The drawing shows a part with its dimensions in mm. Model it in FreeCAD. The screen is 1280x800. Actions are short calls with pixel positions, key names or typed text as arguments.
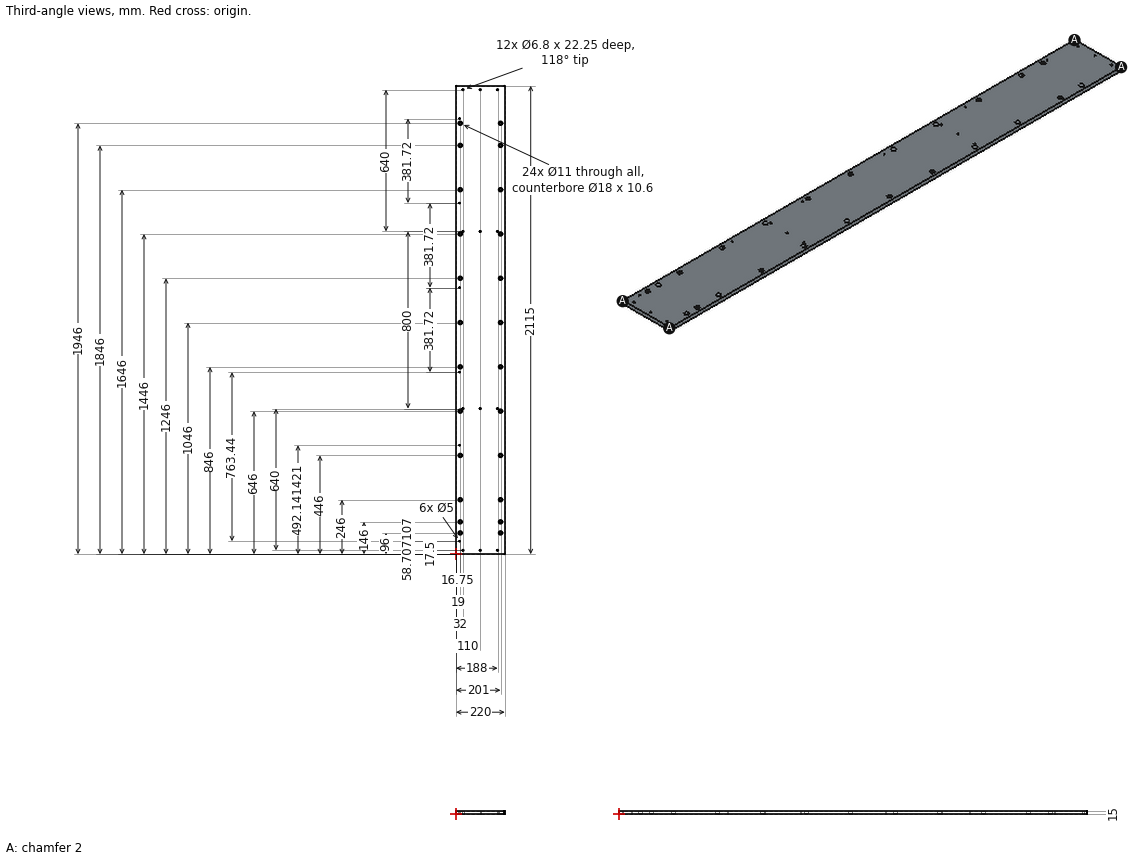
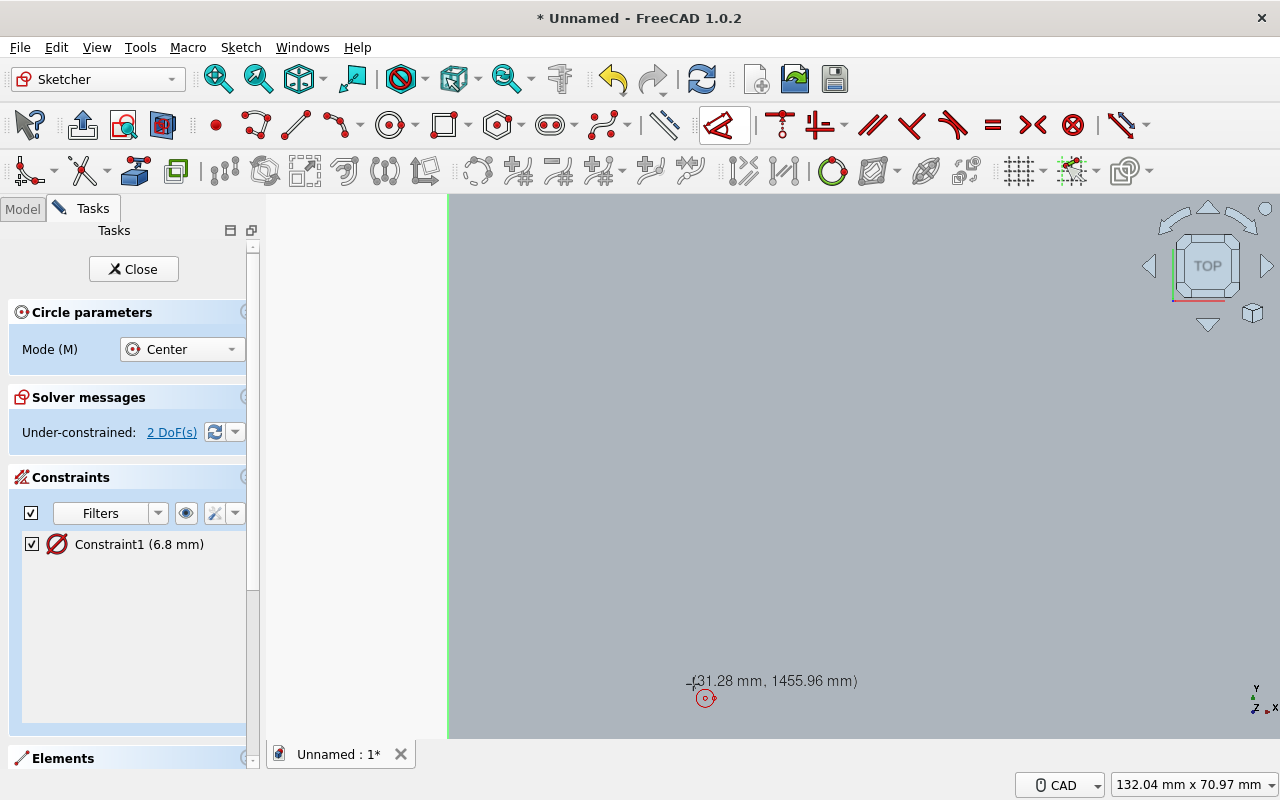
scroll(704, 466, down, 15)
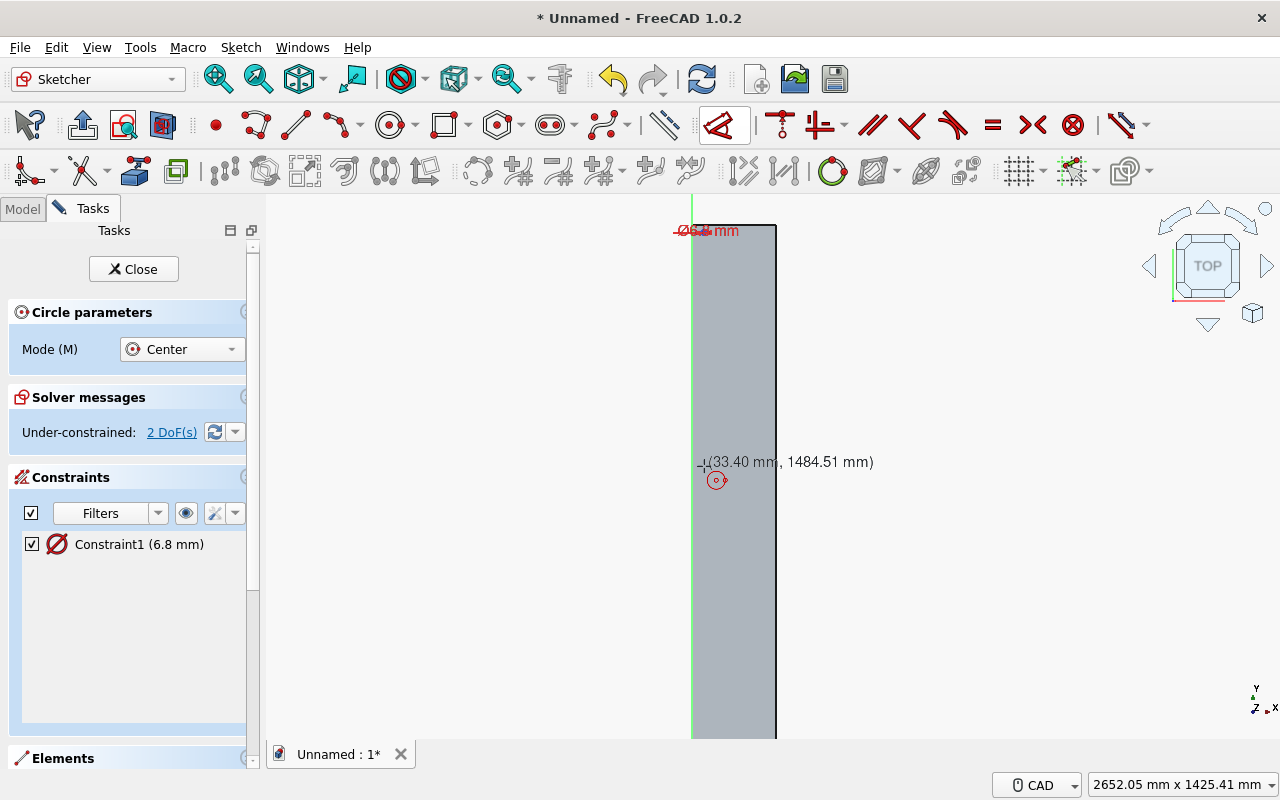
scroll(685, 331, down, 4)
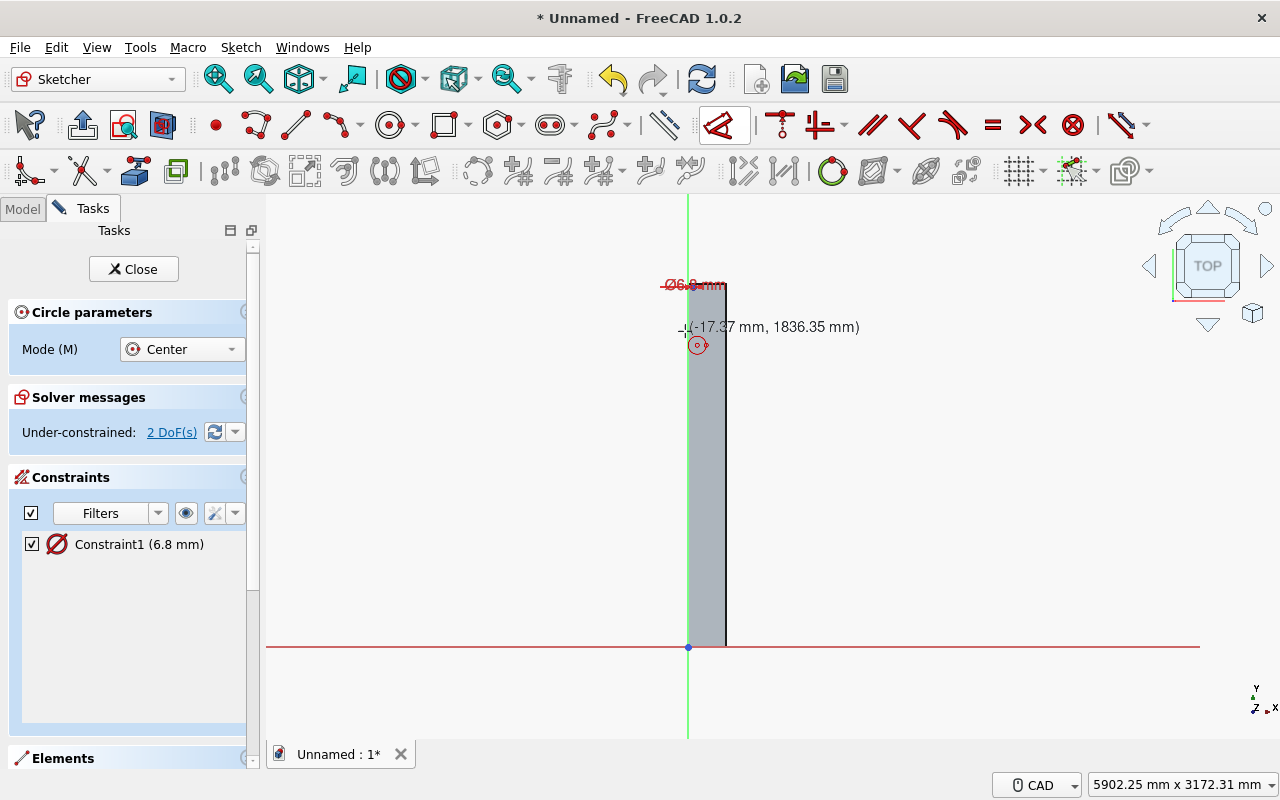
scroll(694, 397, up, 6)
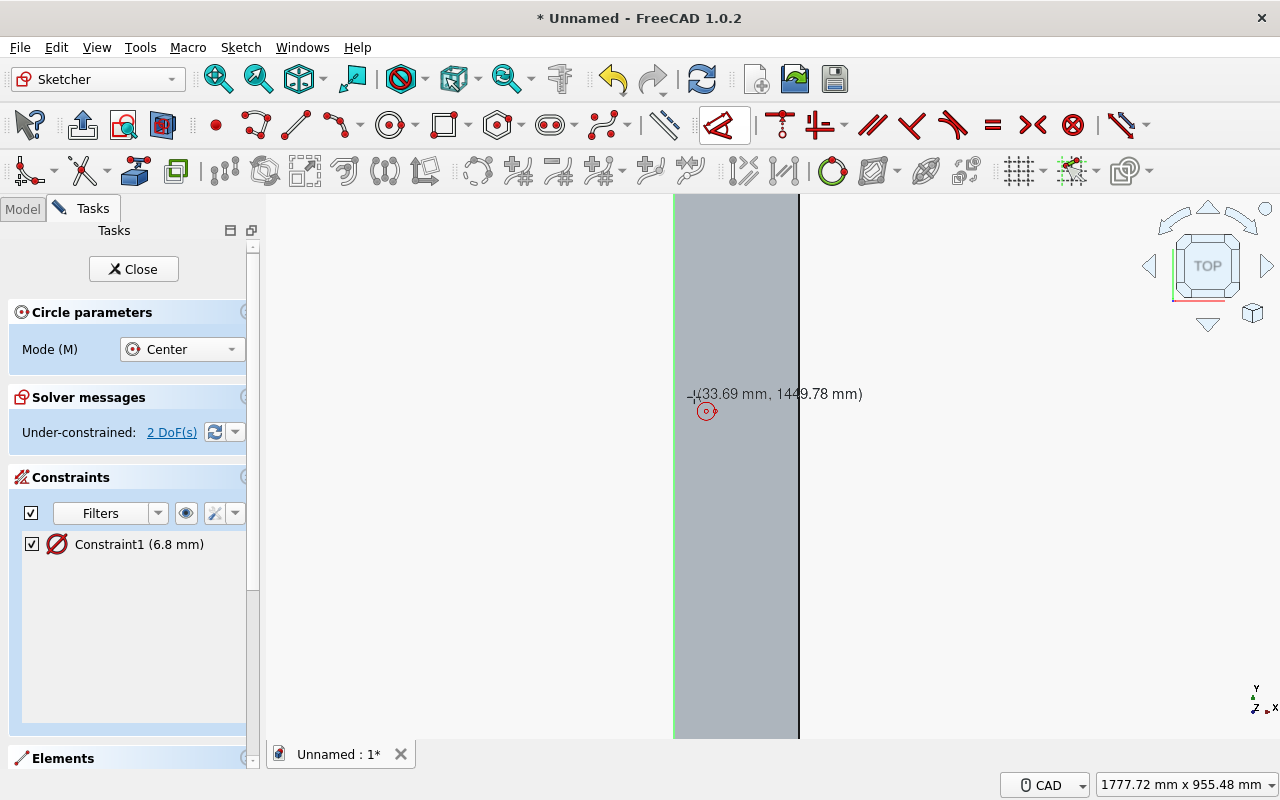
click(692, 395)
move(693, 394)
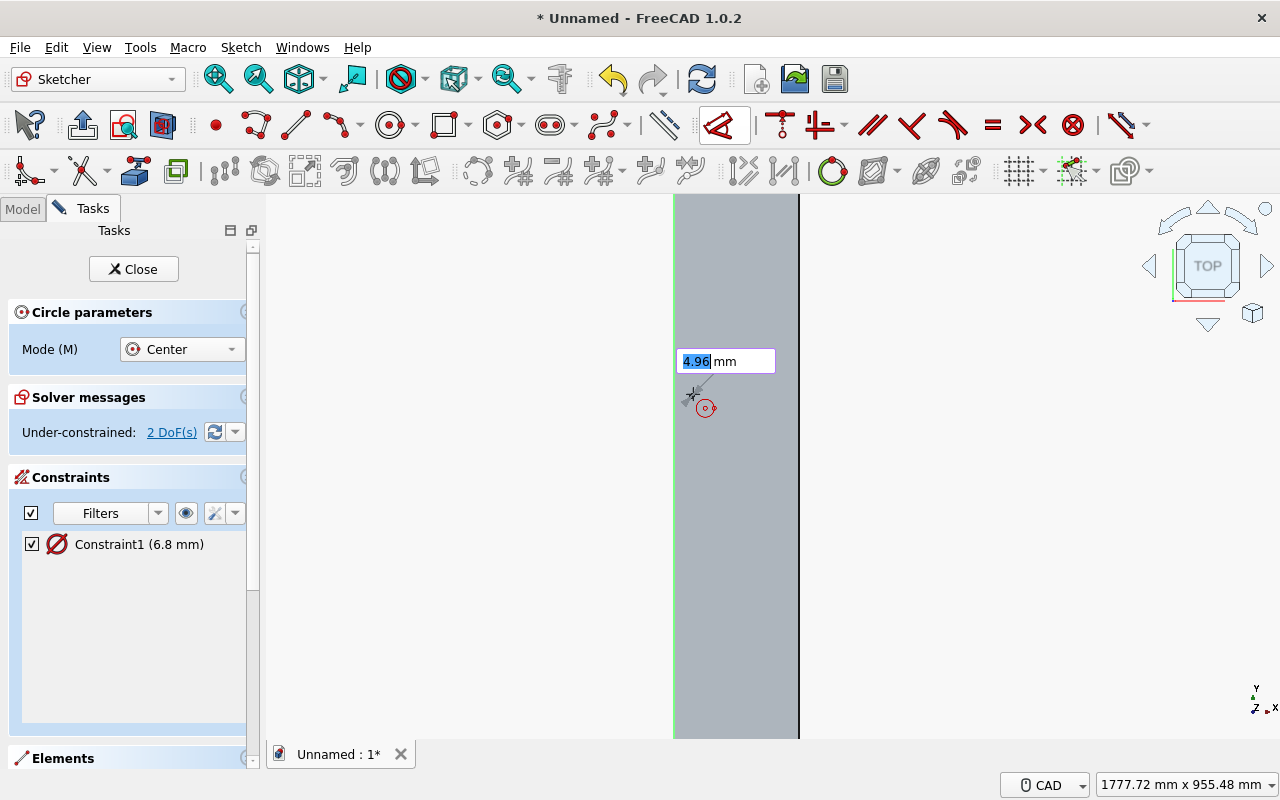
text(6.8)
key(Return)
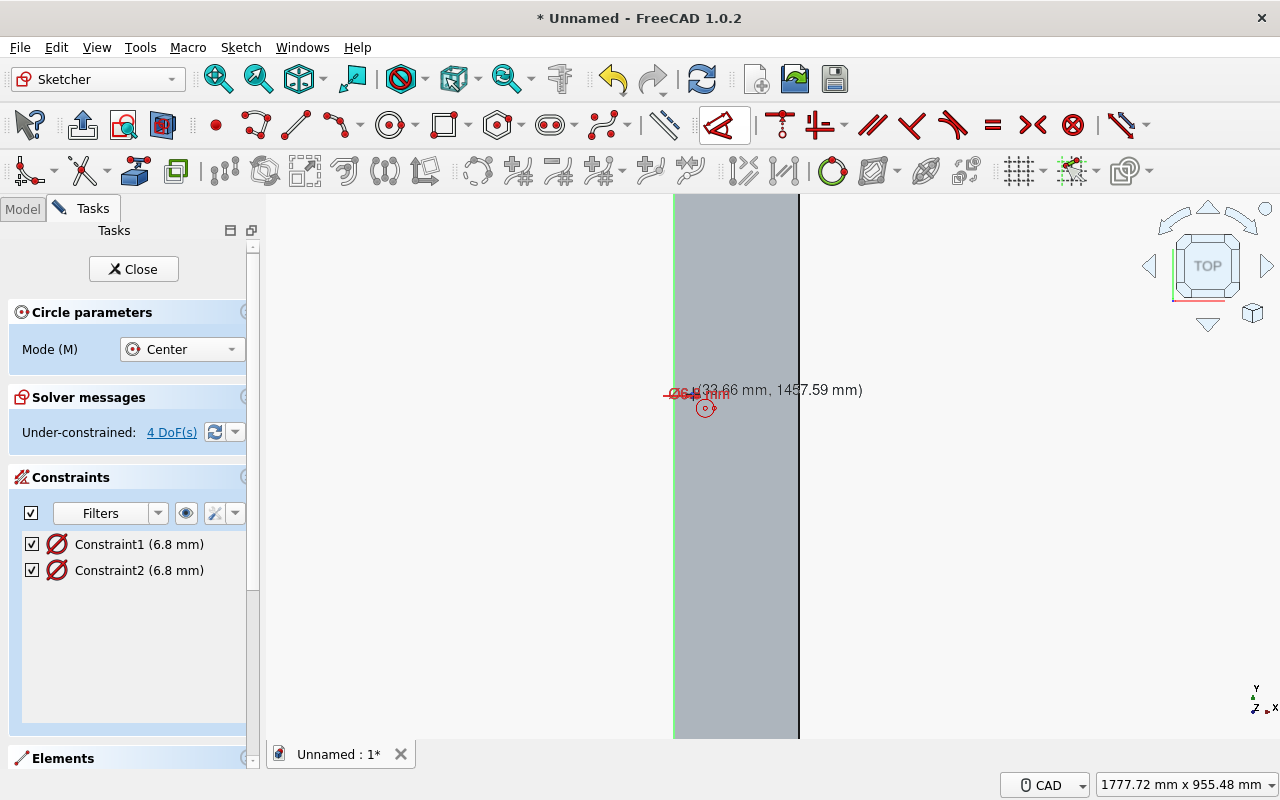
scroll(694, 397, down, 6)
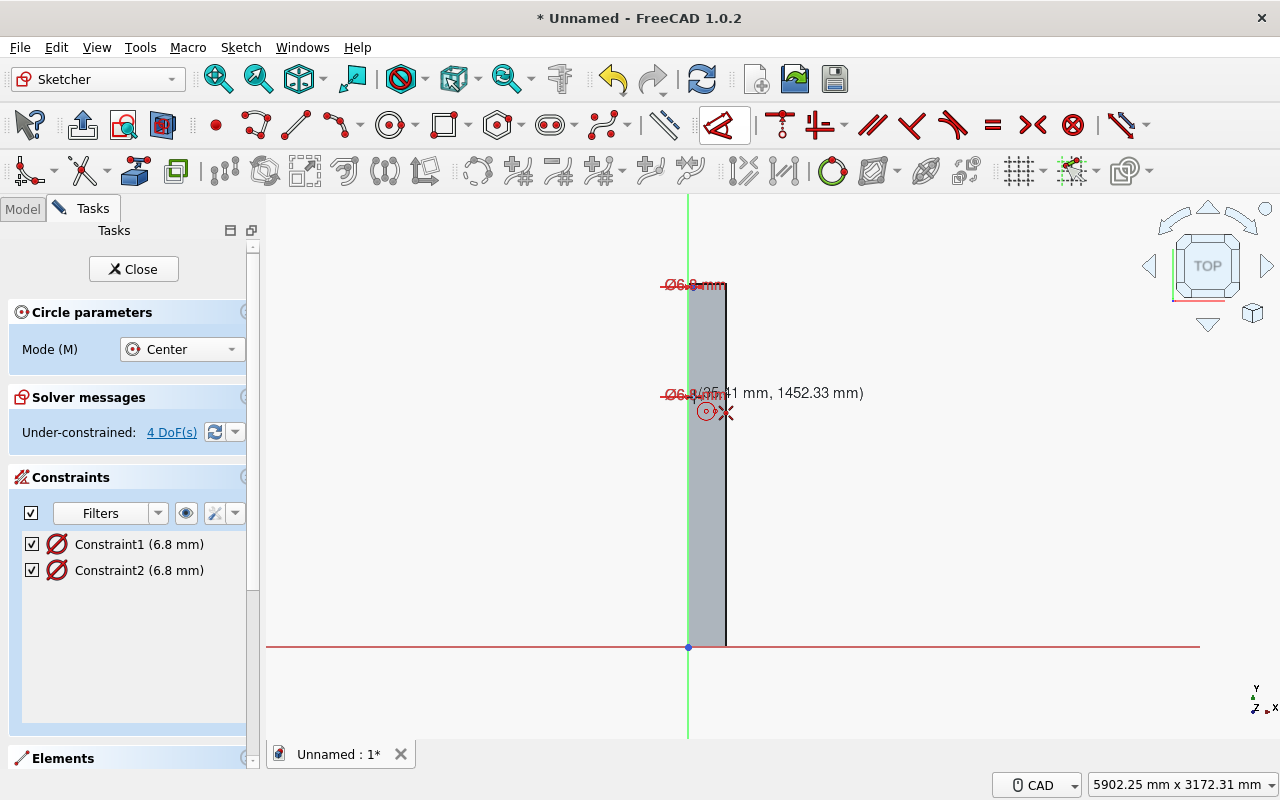
scroll(694, 534, up, 19)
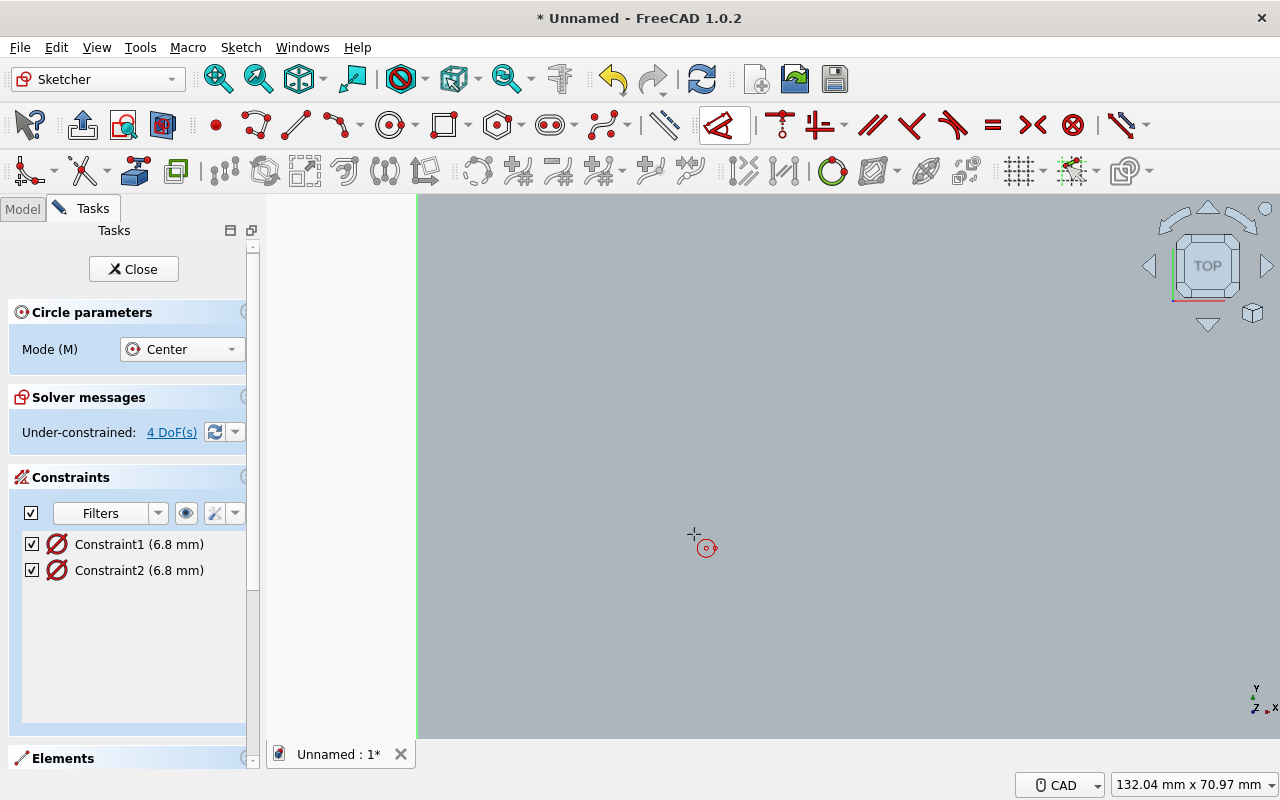
scroll(704, 466, down, 15)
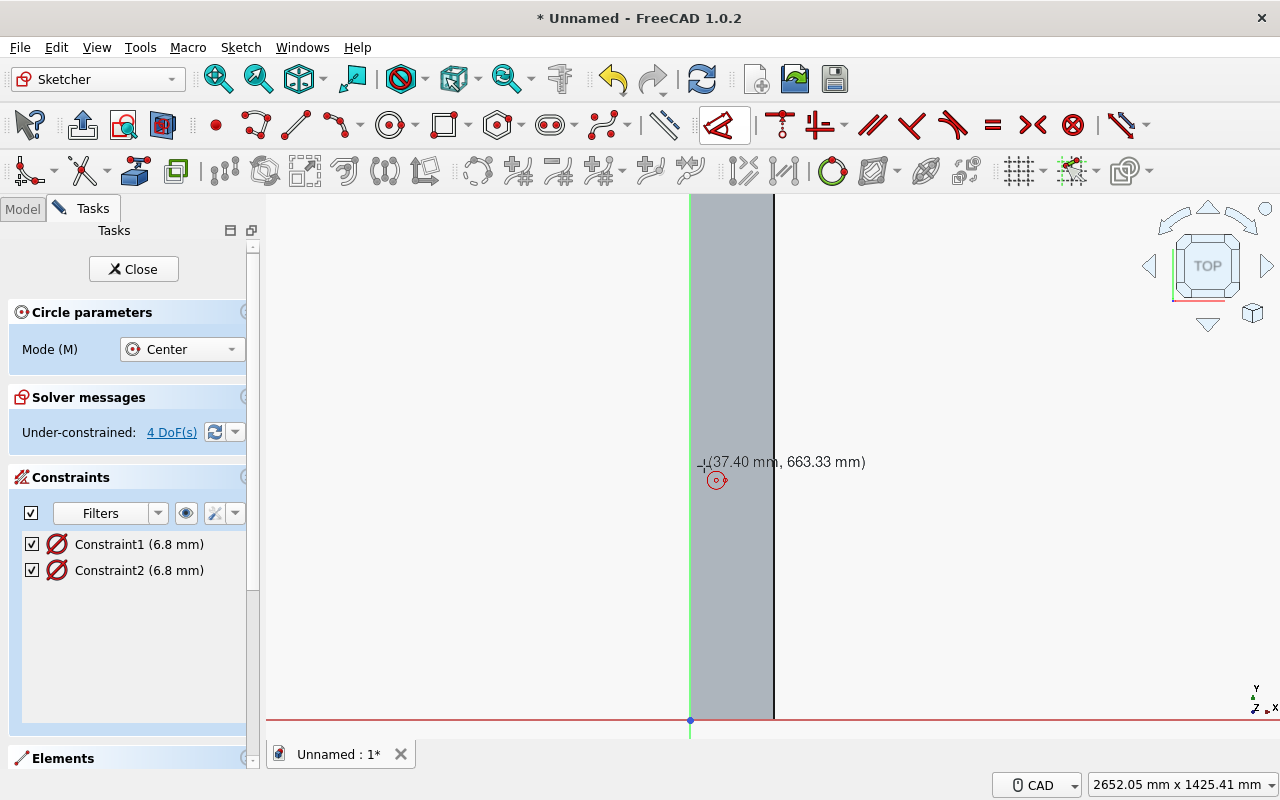
scroll(686, 587, down, 4)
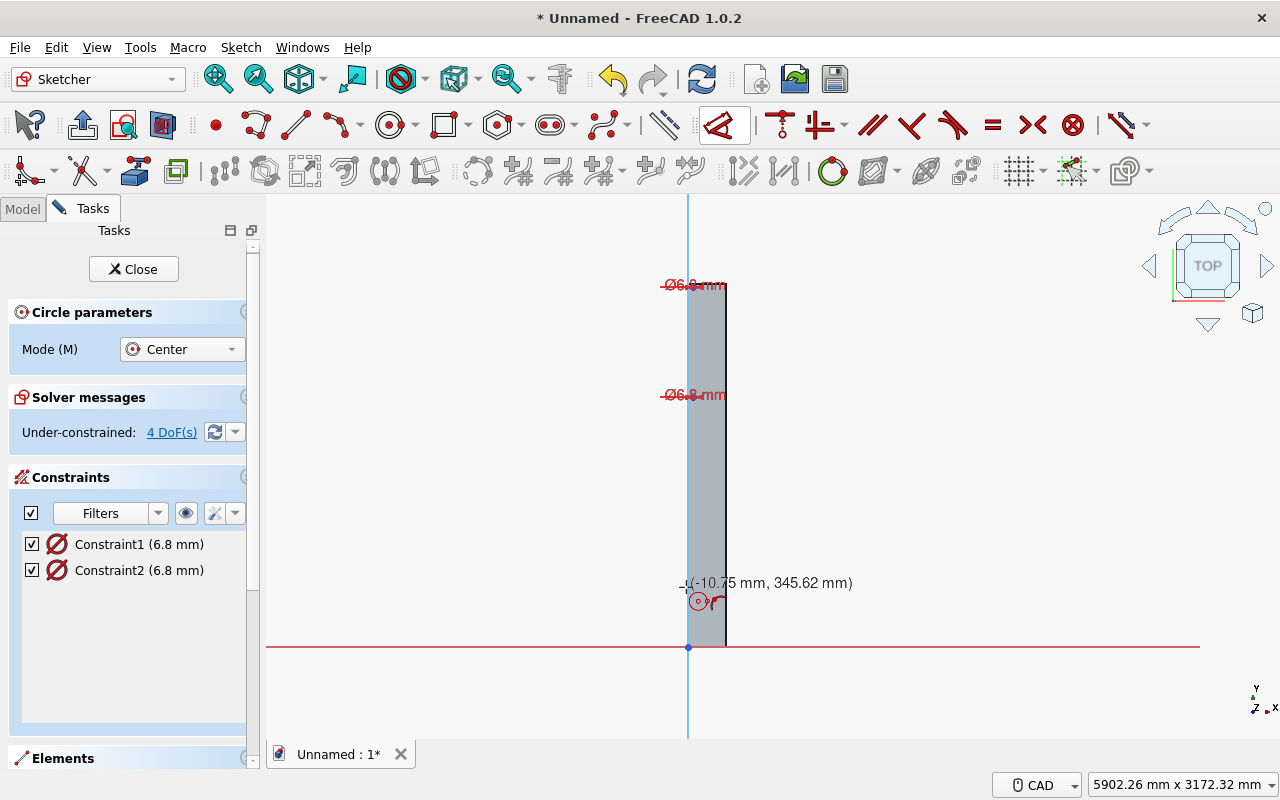
scroll(694, 534, up, 6)